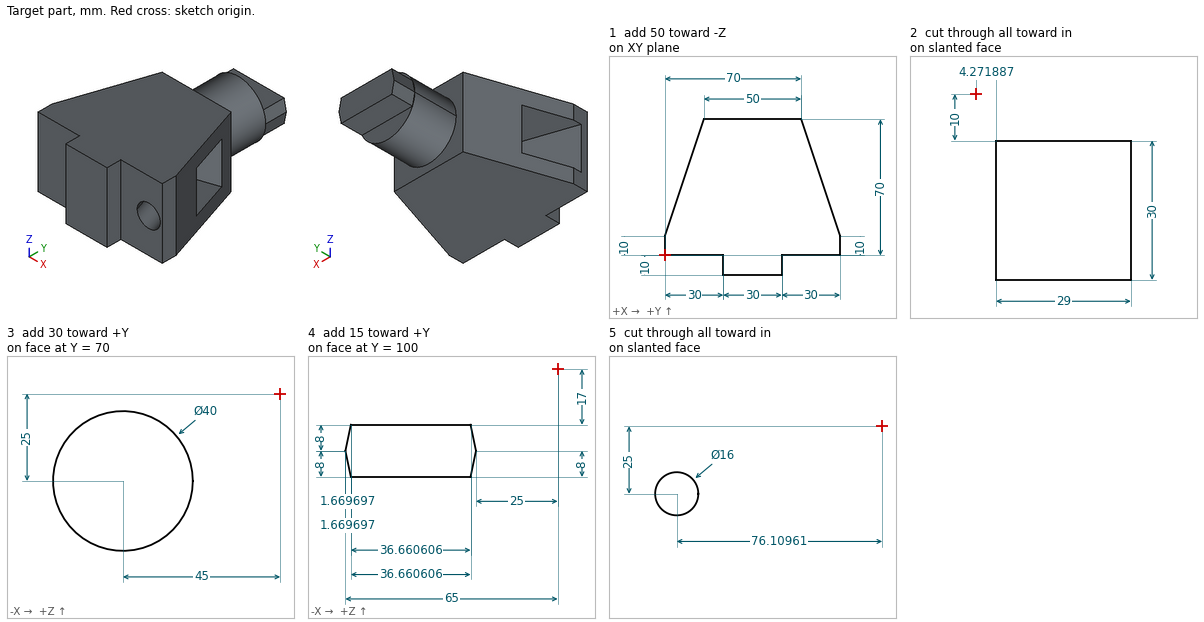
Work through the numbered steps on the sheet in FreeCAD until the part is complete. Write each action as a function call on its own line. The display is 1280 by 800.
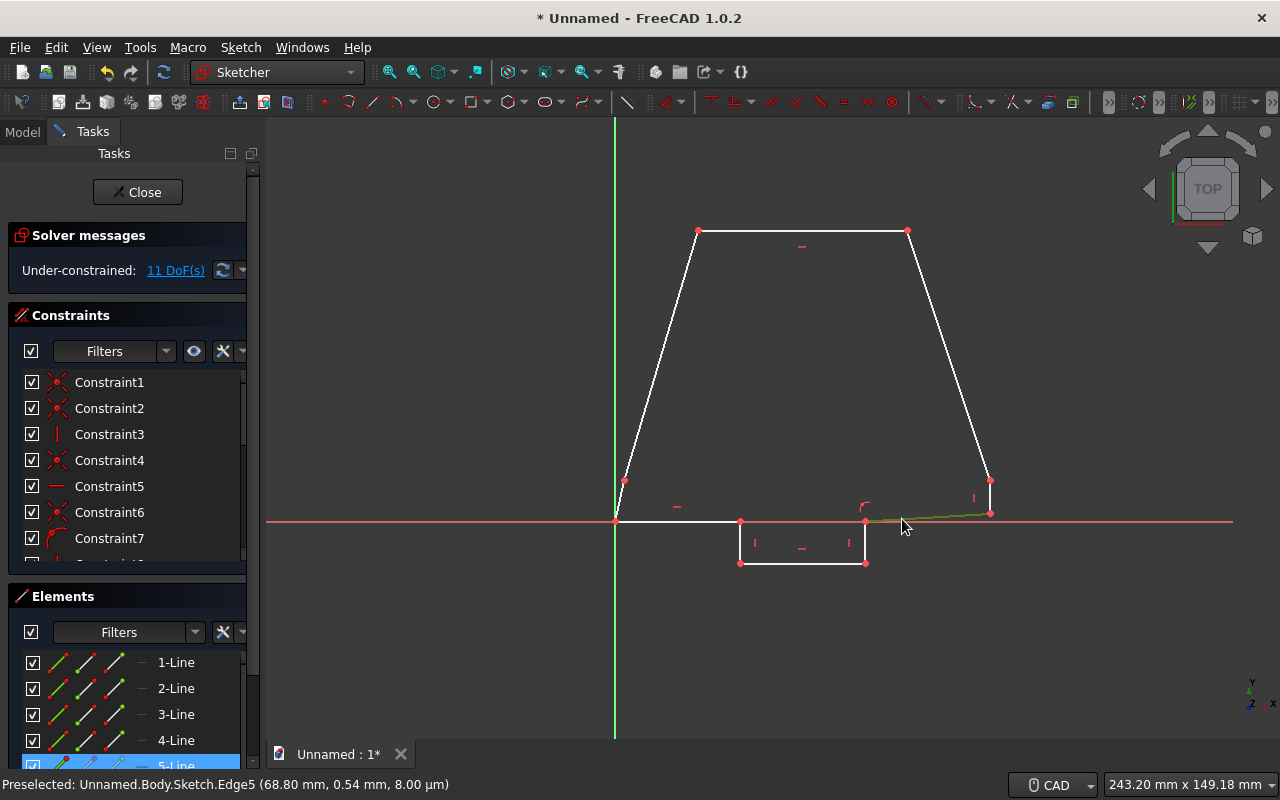
key(h)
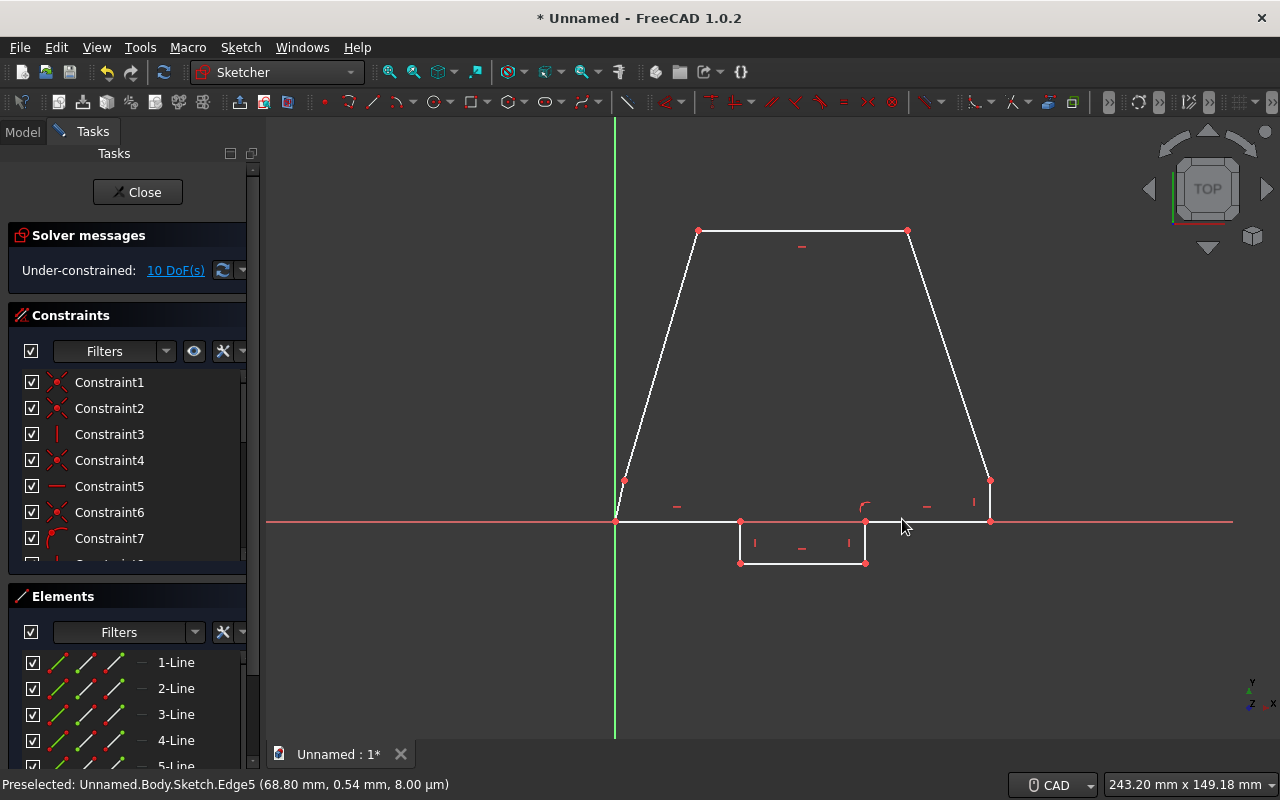
click(618, 509)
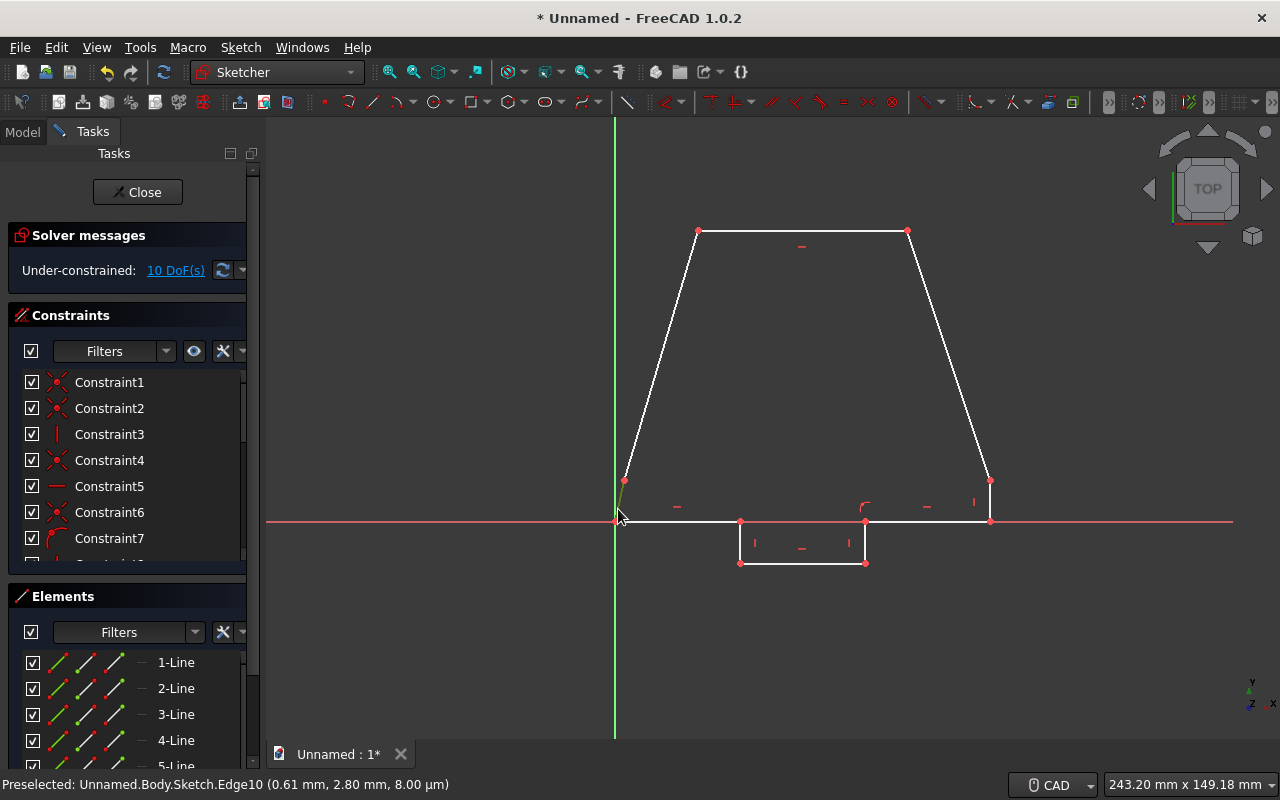
key(v)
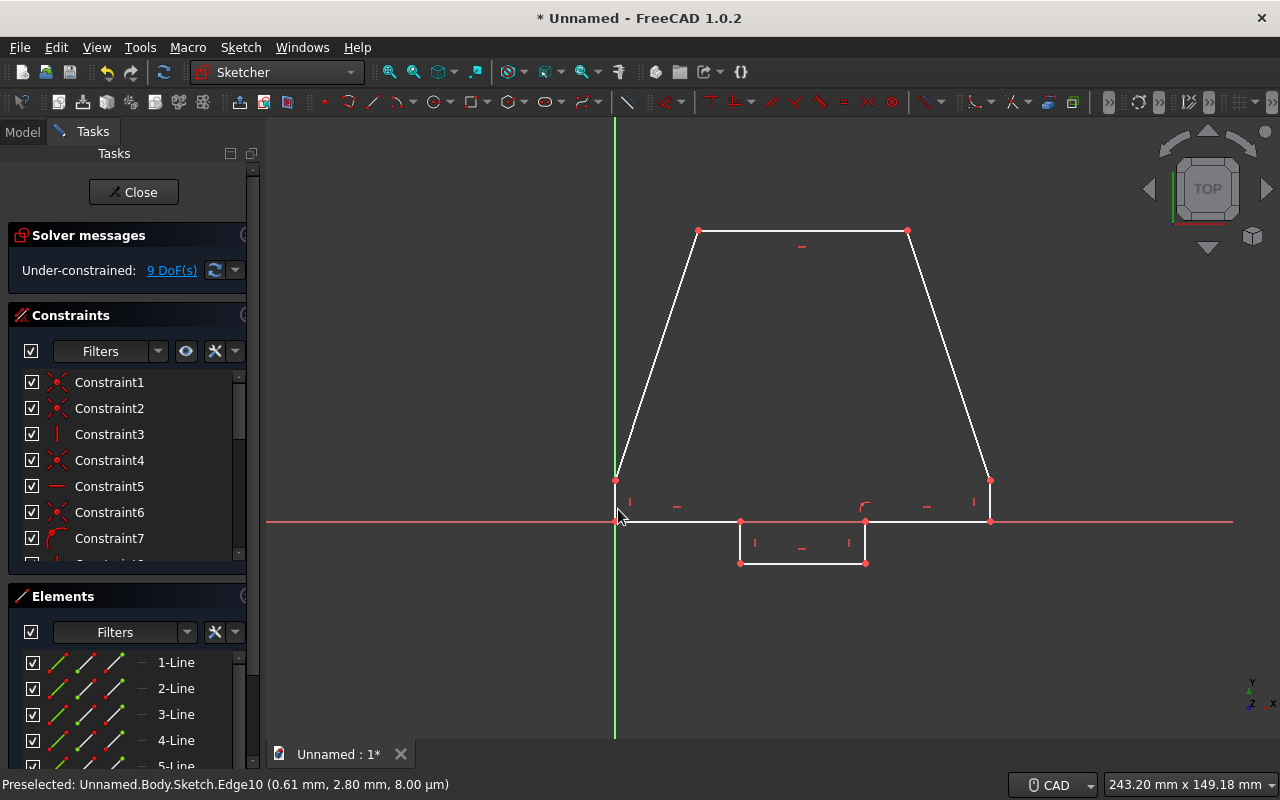
key(d)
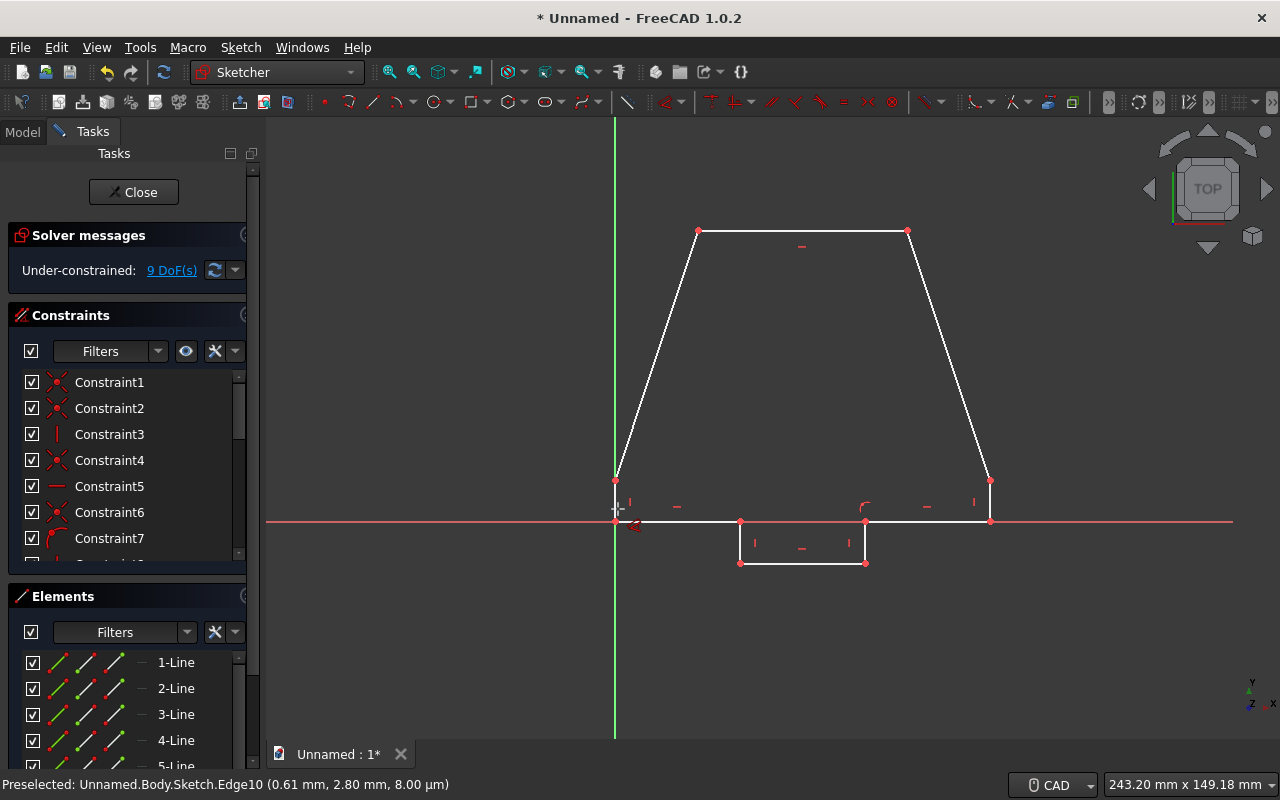
click(653, 522)
click(678, 556)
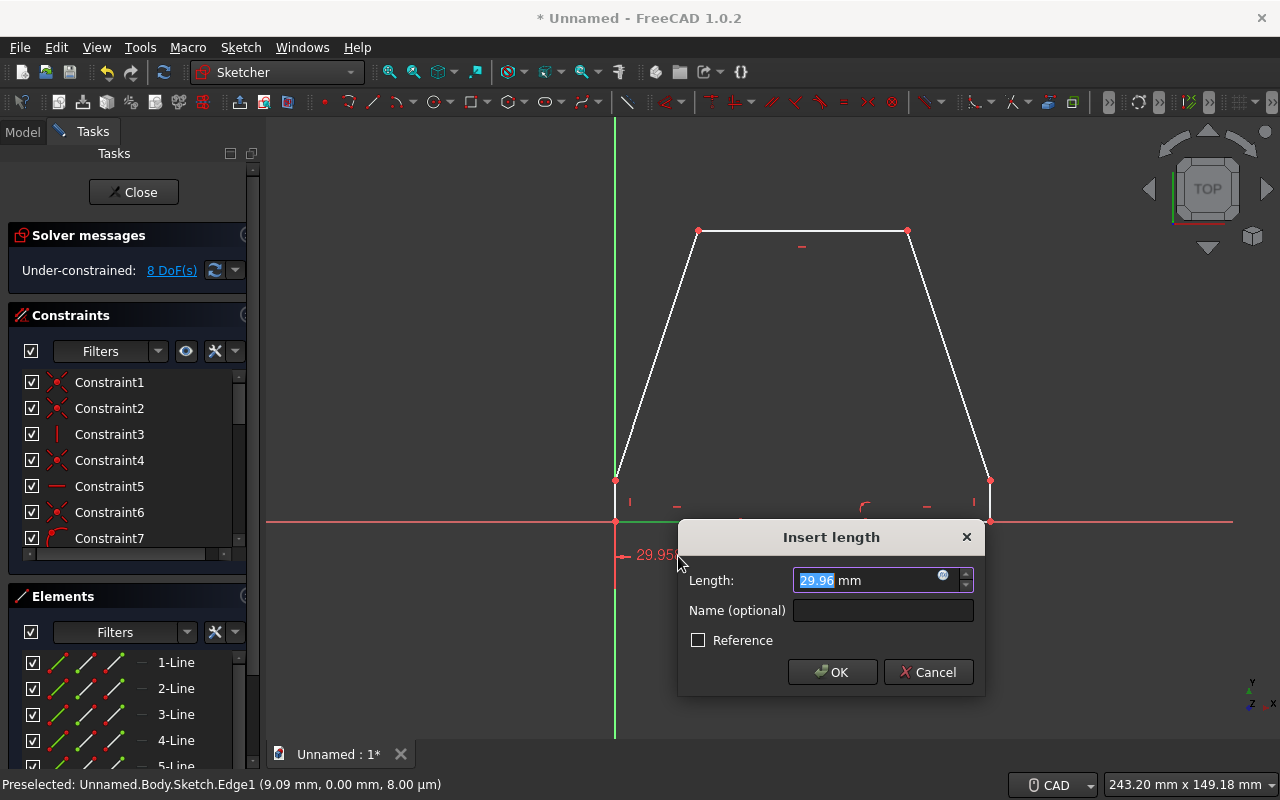
text(30)
key(Return)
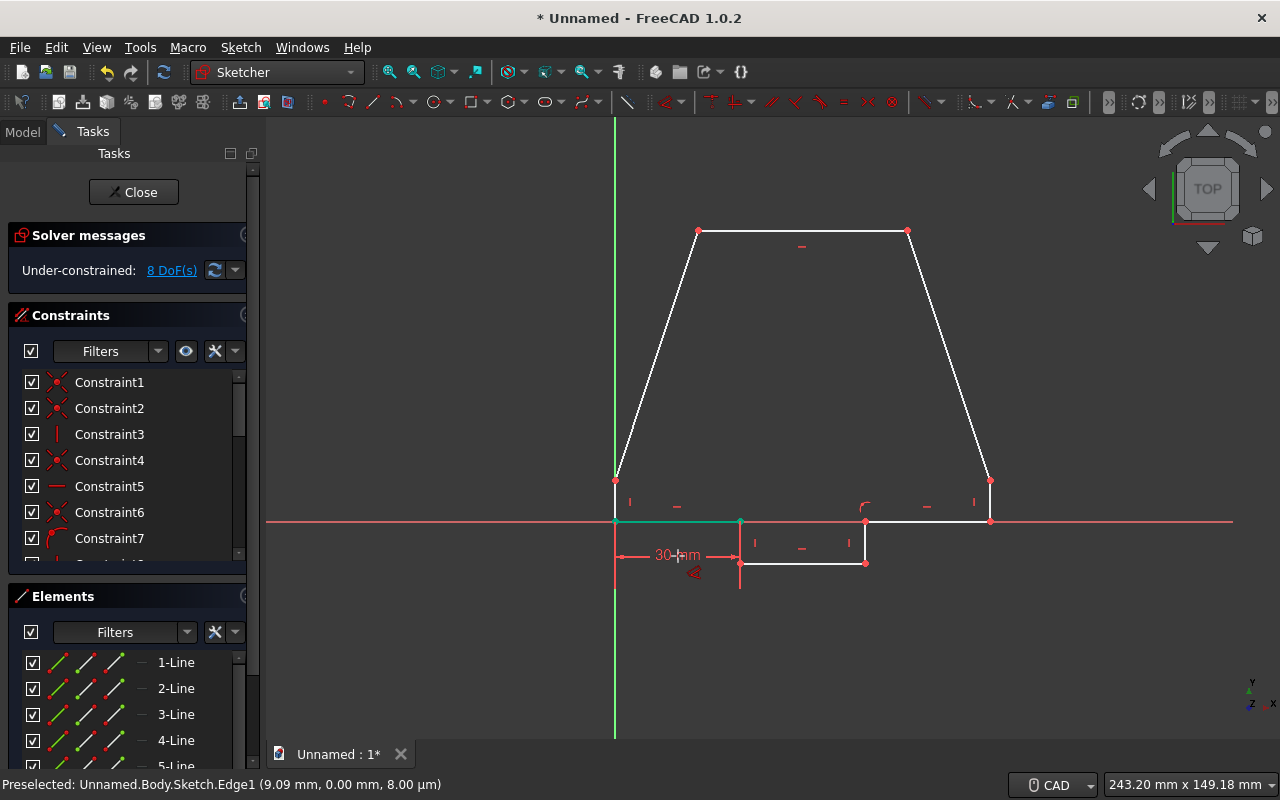
click(740, 534)
click(774, 543)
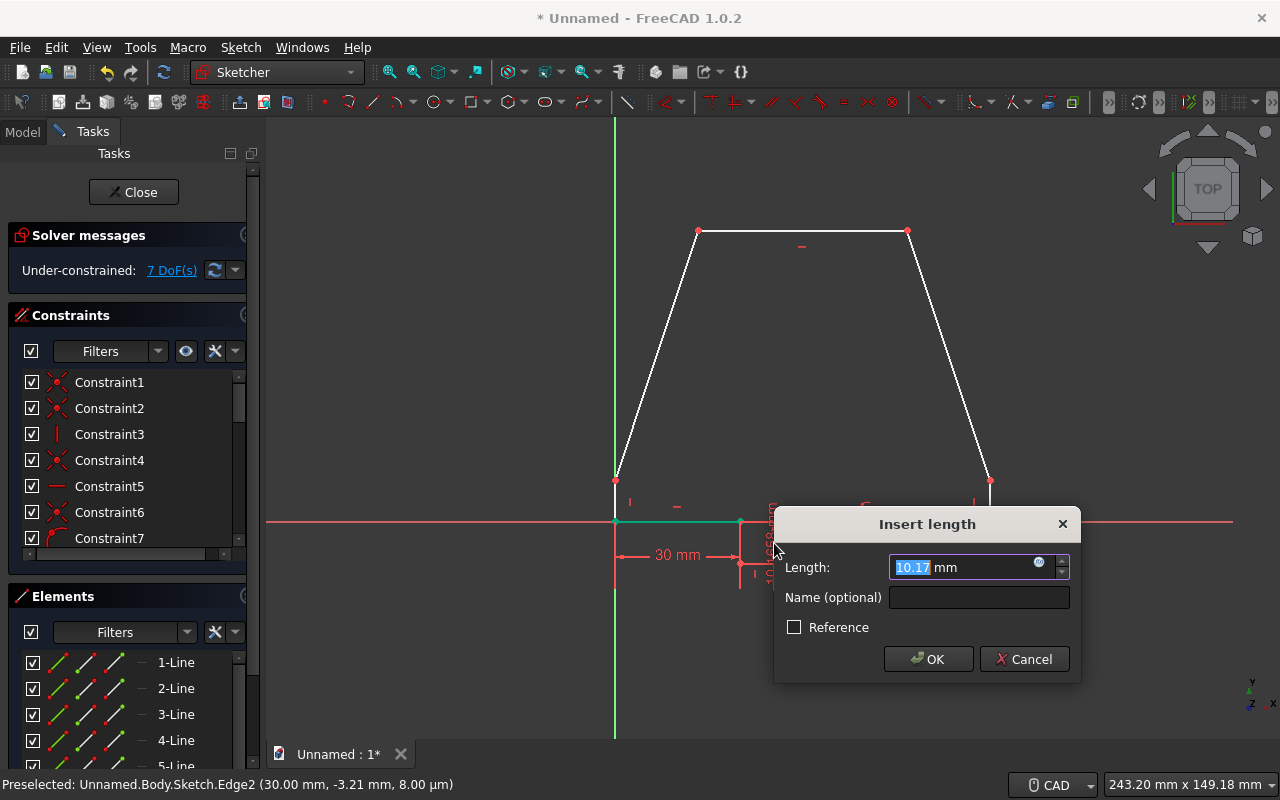
text(10)
key(Return)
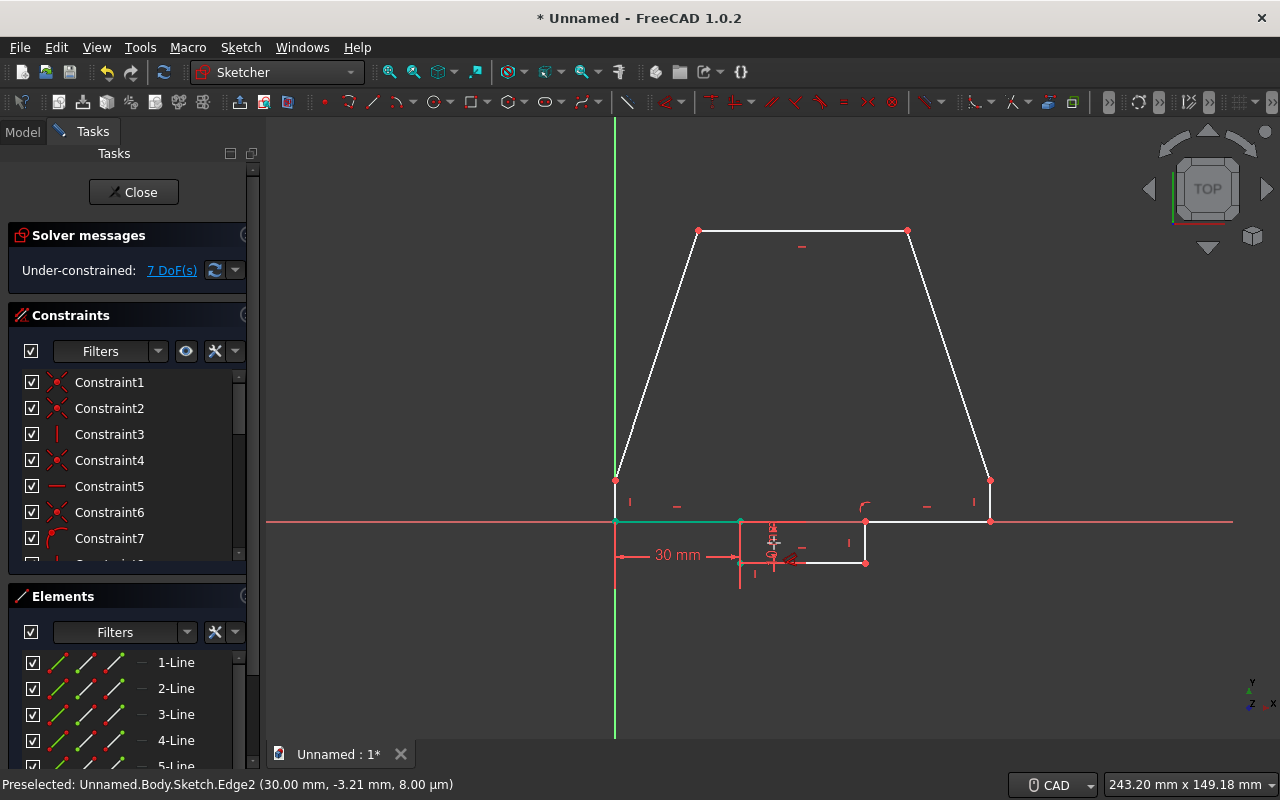
click(778, 563)
click(803, 597)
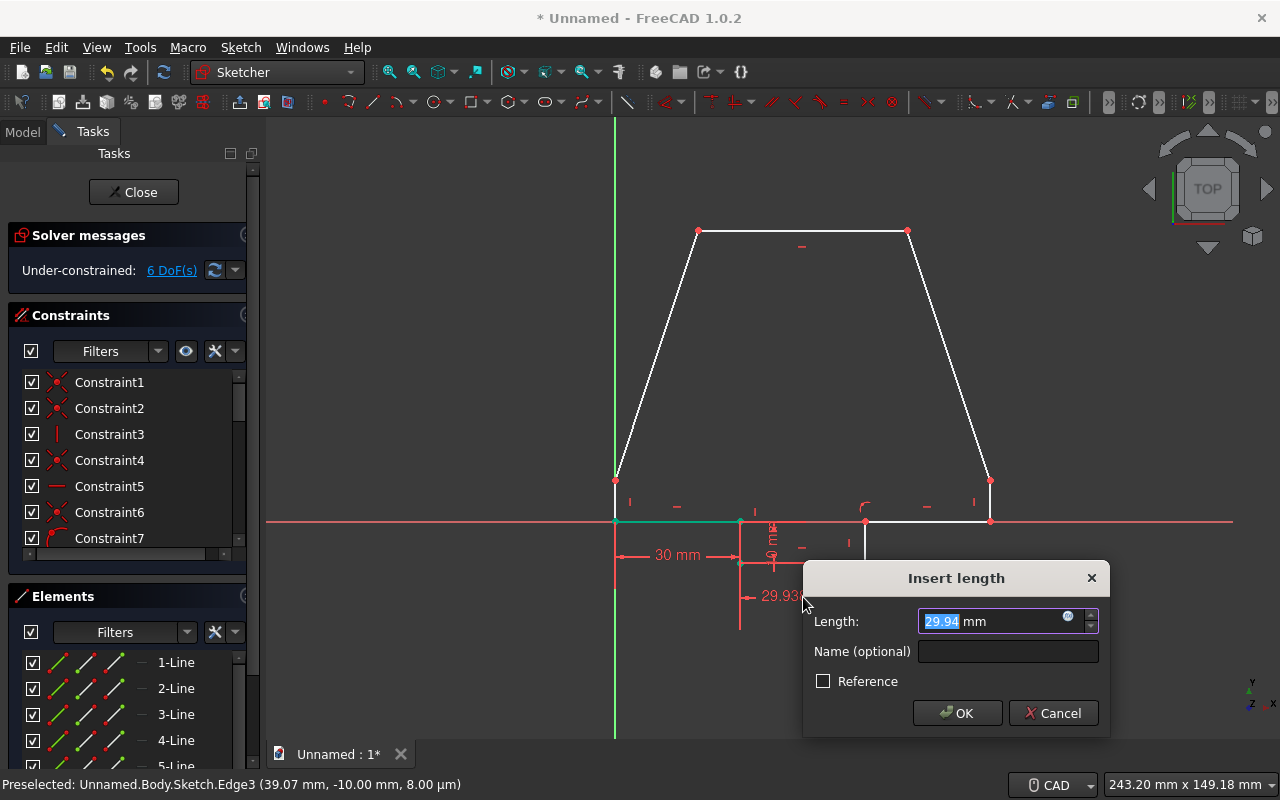
text(30)
key(Return)